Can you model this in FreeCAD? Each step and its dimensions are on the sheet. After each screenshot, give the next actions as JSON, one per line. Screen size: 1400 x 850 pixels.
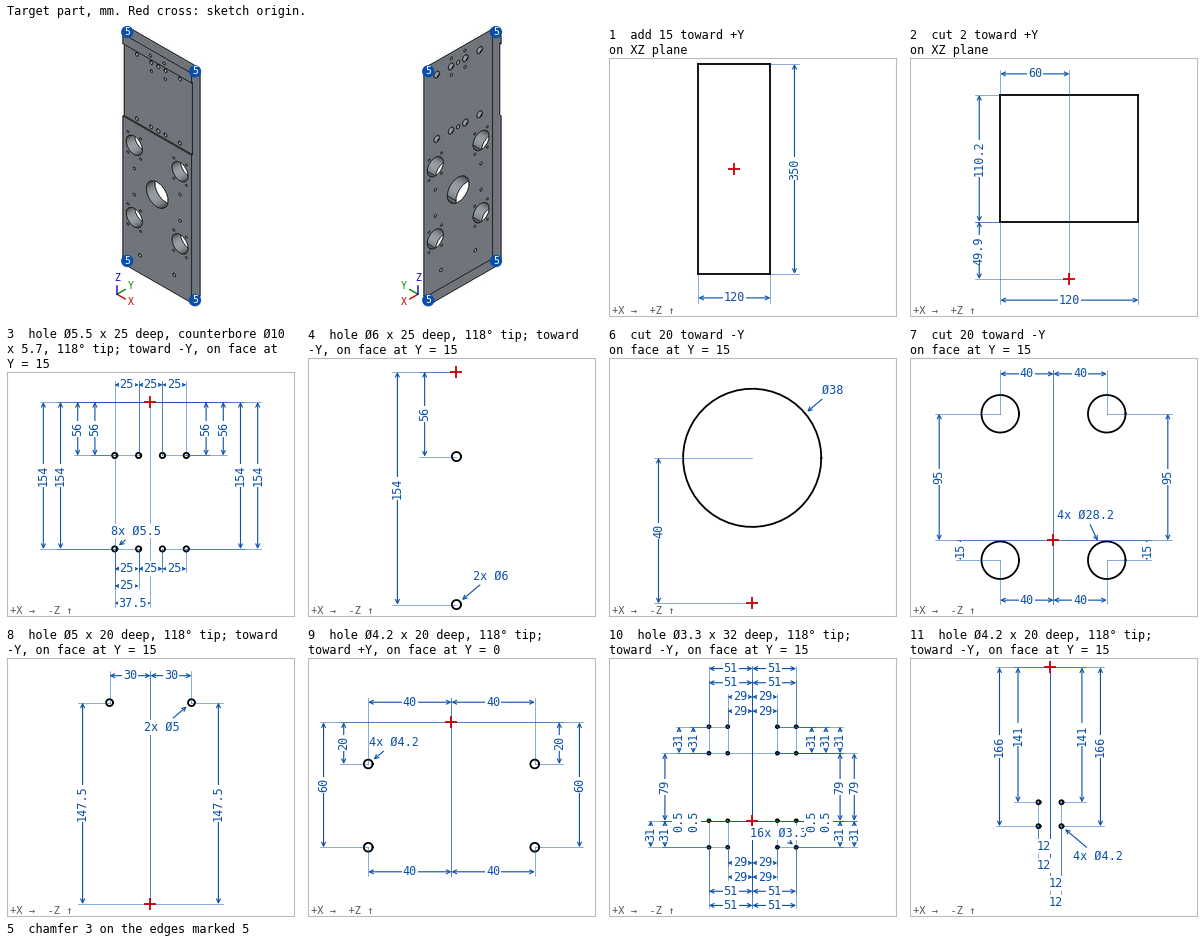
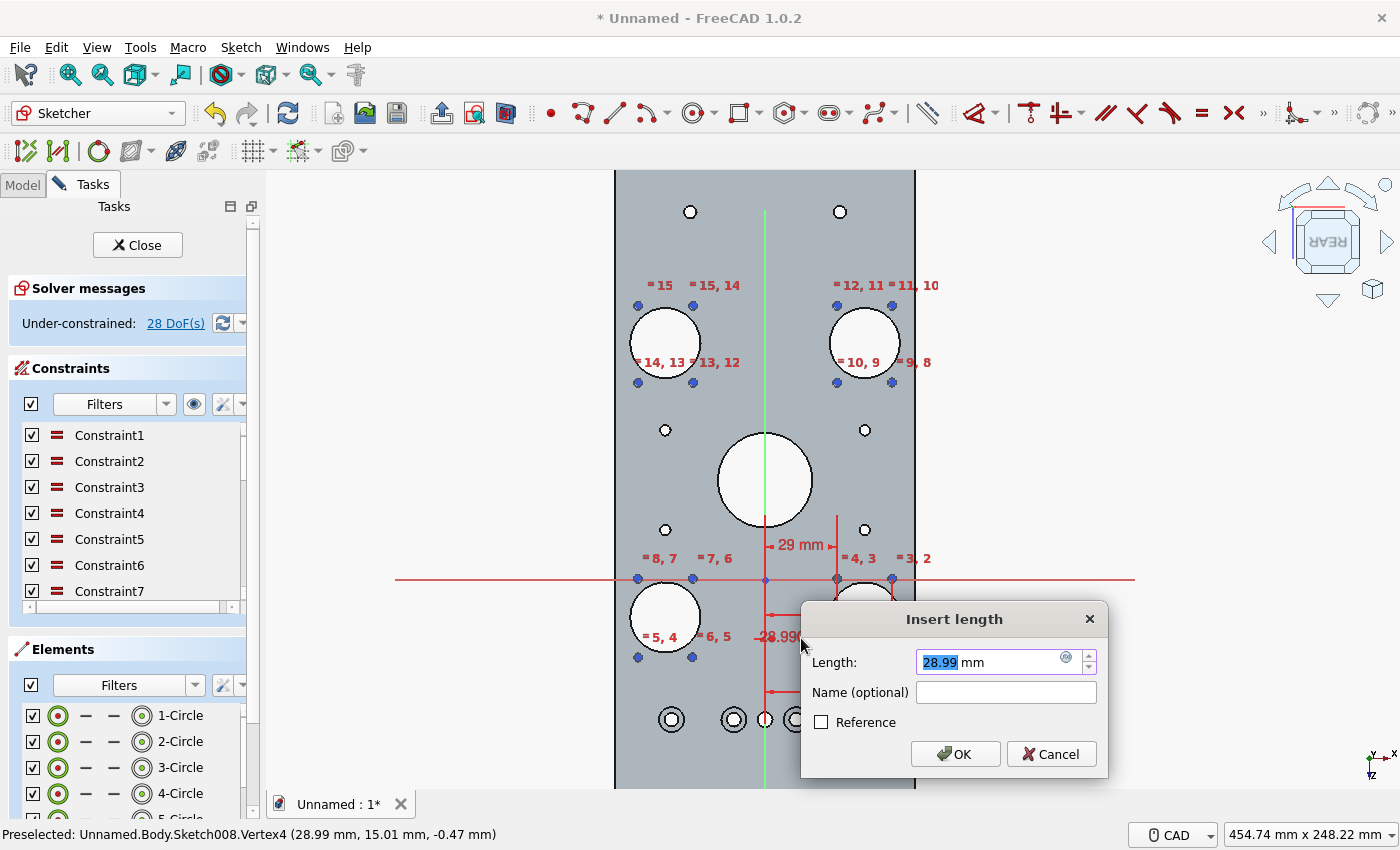
{"action": "type", "text": "29"}
{"action": "key", "text": "Return"}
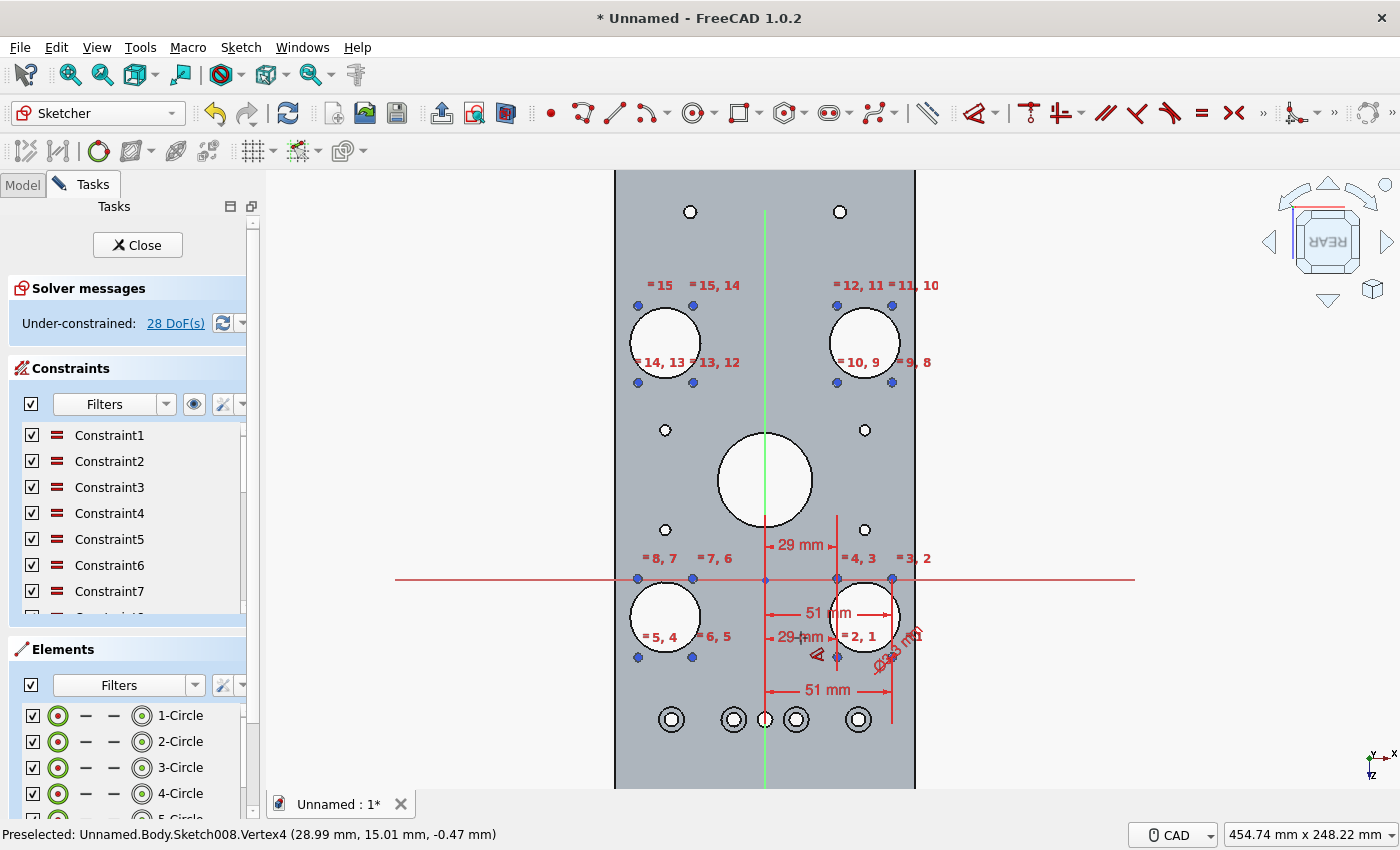
{"action": "left_click", "coordinate": [638, 657]}
{"action": "left_click", "coordinate": [702, 691]}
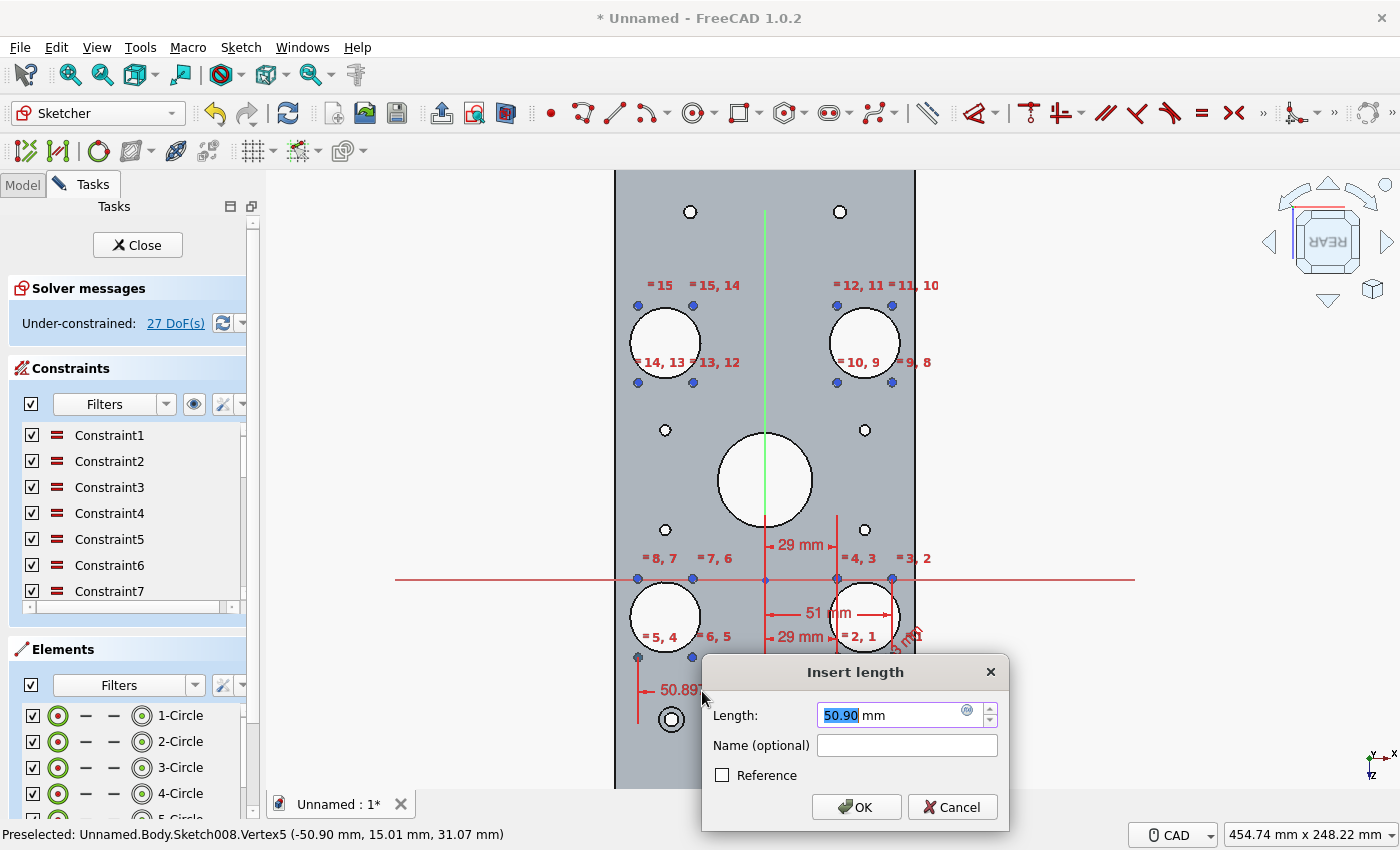
{"action": "type", "text": "51"}
{"action": "key", "text": "Return"}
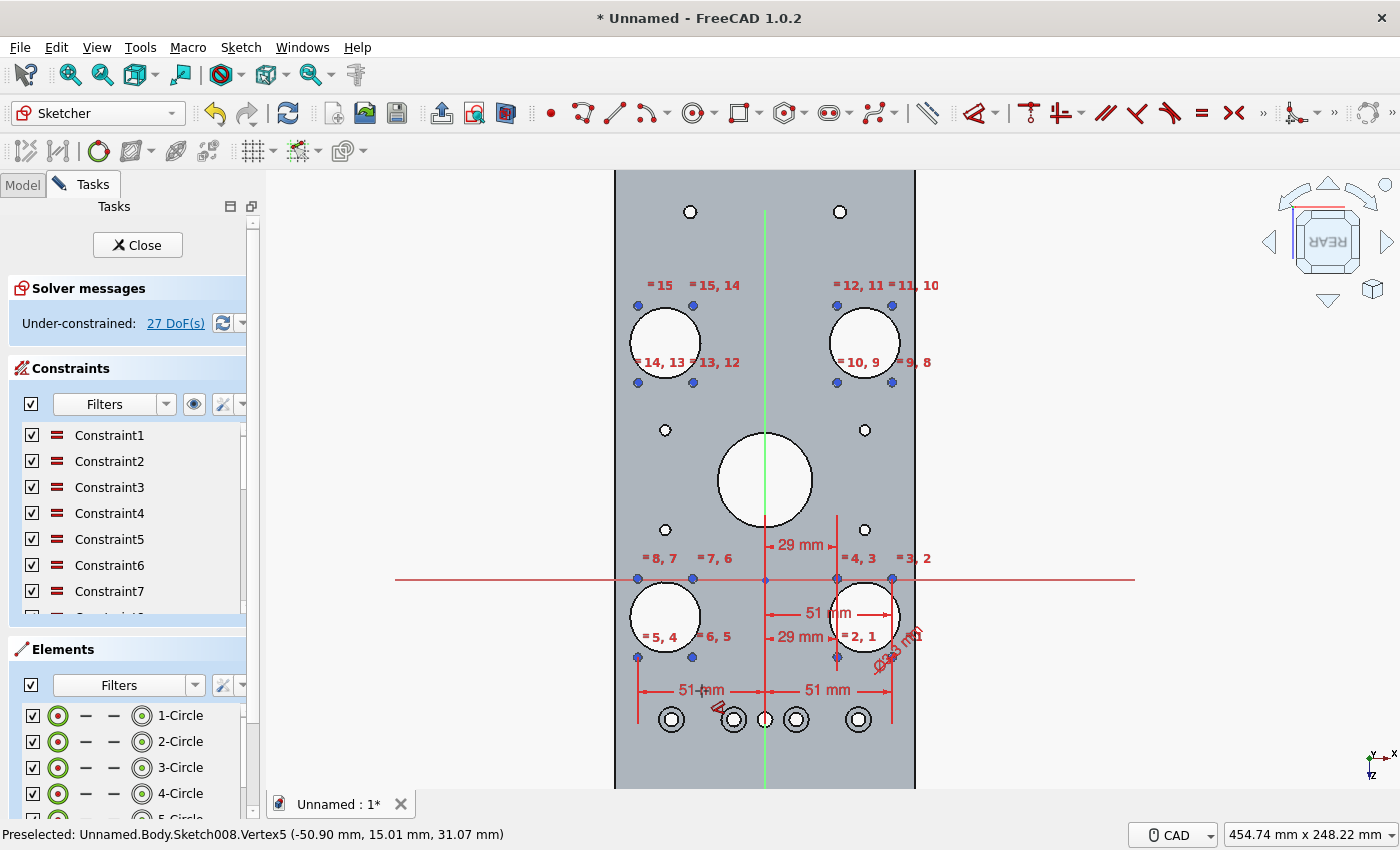
{"action": "left_click", "coordinate": [692, 657]}
{"action": "left_click", "coordinate": [729, 546]}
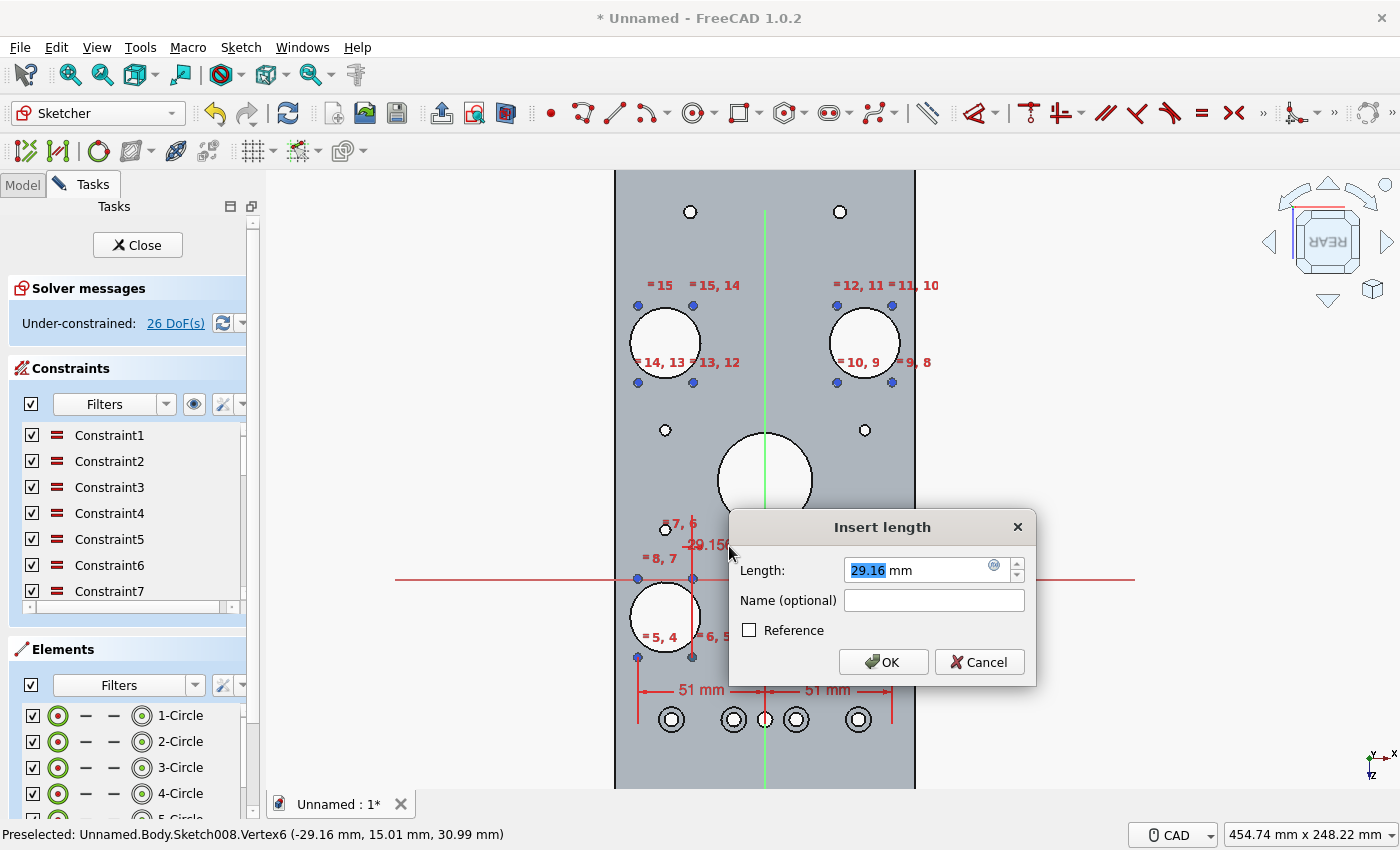
{"action": "type", "text": "29"}
{"action": "key", "text": "Return"}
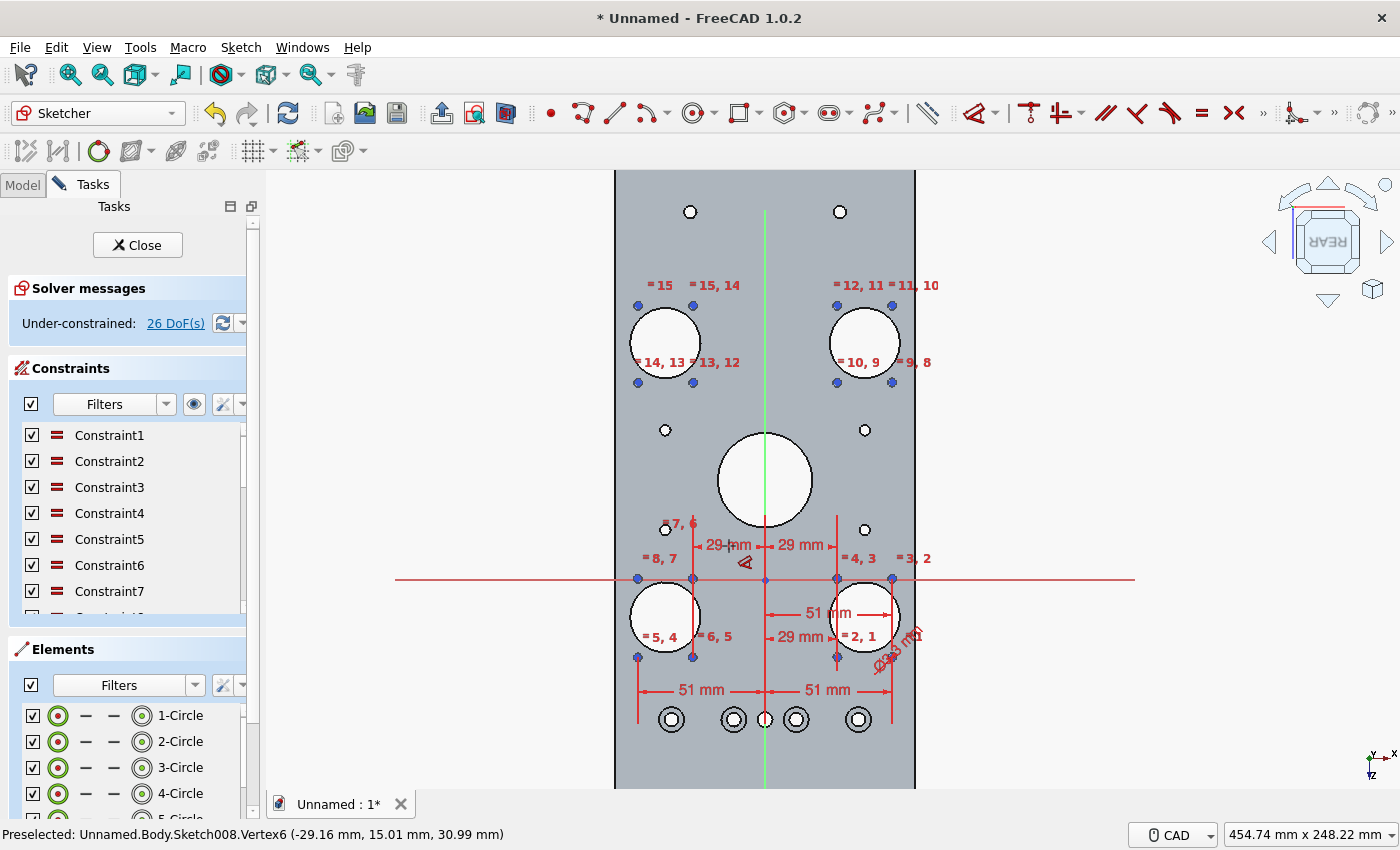
{"action": "left_click", "coordinate": [693, 579]}
{"action": "left_click", "coordinate": [729, 614]}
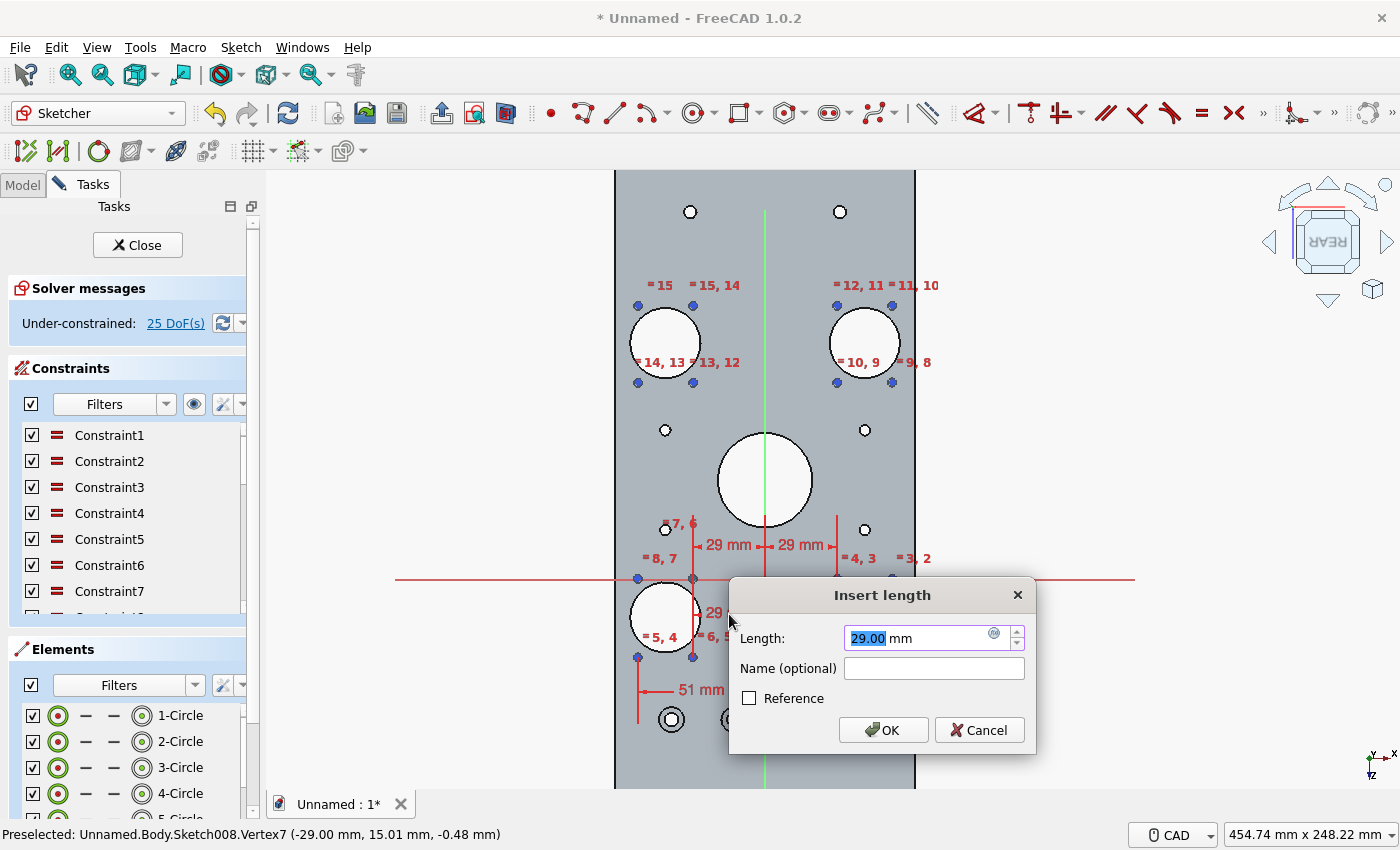
{"action": "type", "text": "29"}
{"action": "key", "text": "Return"}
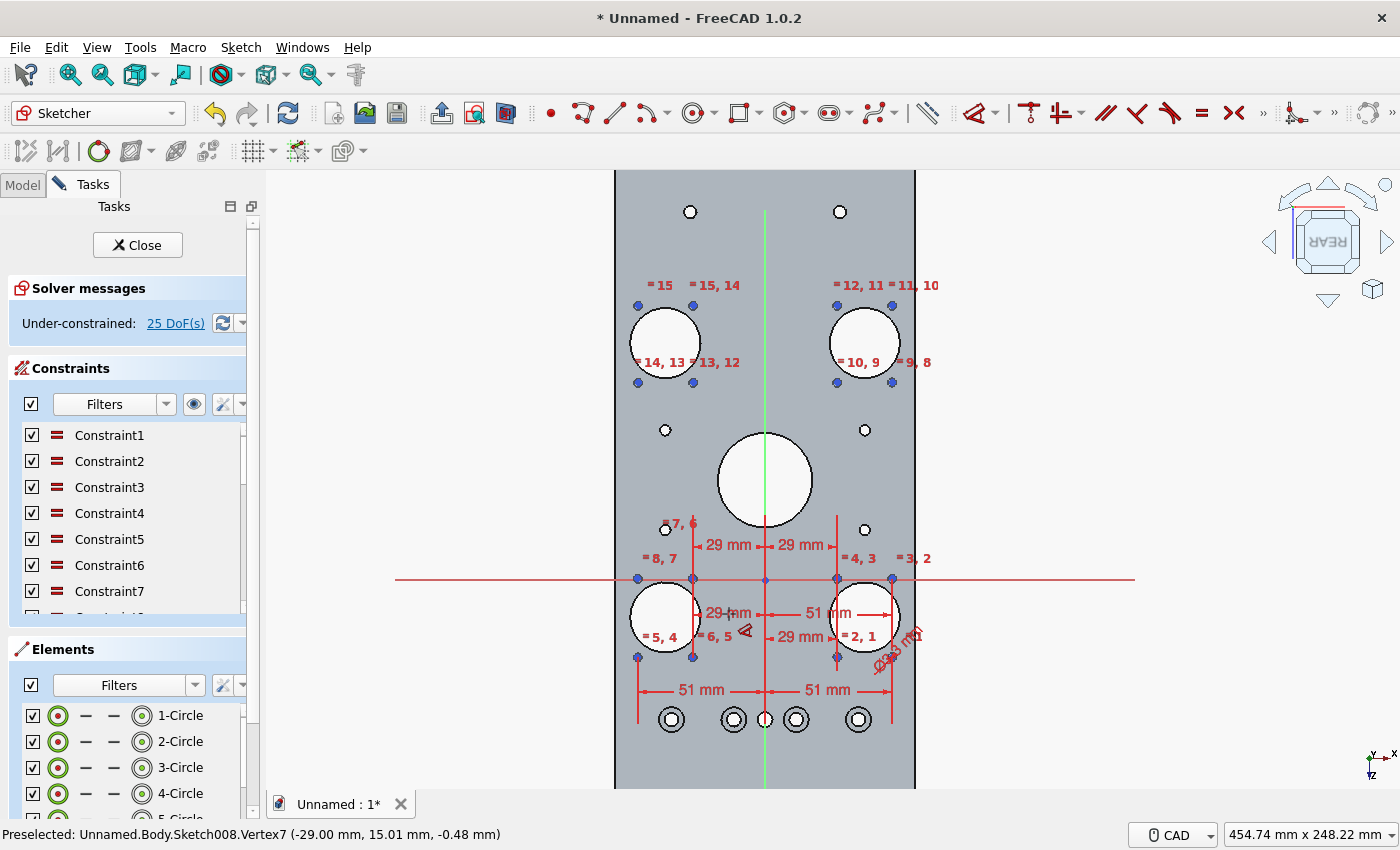
{"action": "left_click", "coordinate": [638, 579]}
{"action": "left_click", "coordinate": [657, 614]}